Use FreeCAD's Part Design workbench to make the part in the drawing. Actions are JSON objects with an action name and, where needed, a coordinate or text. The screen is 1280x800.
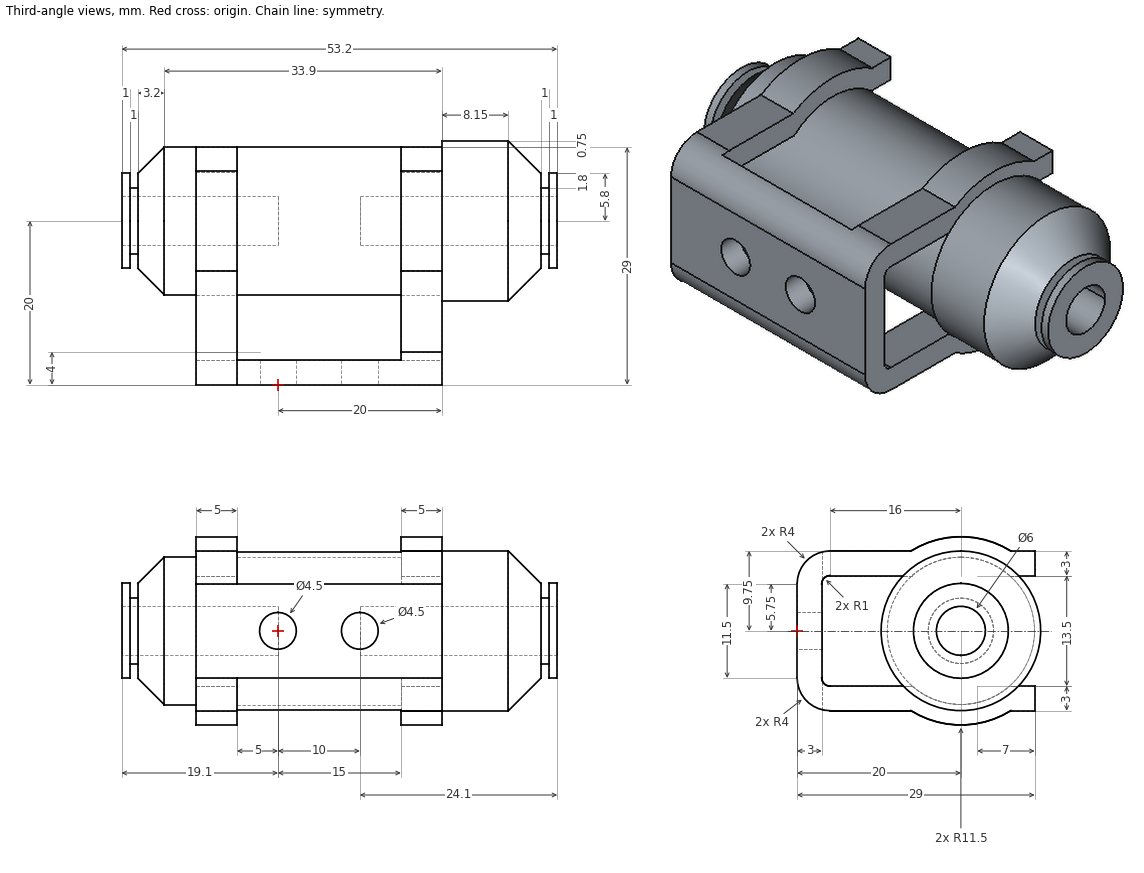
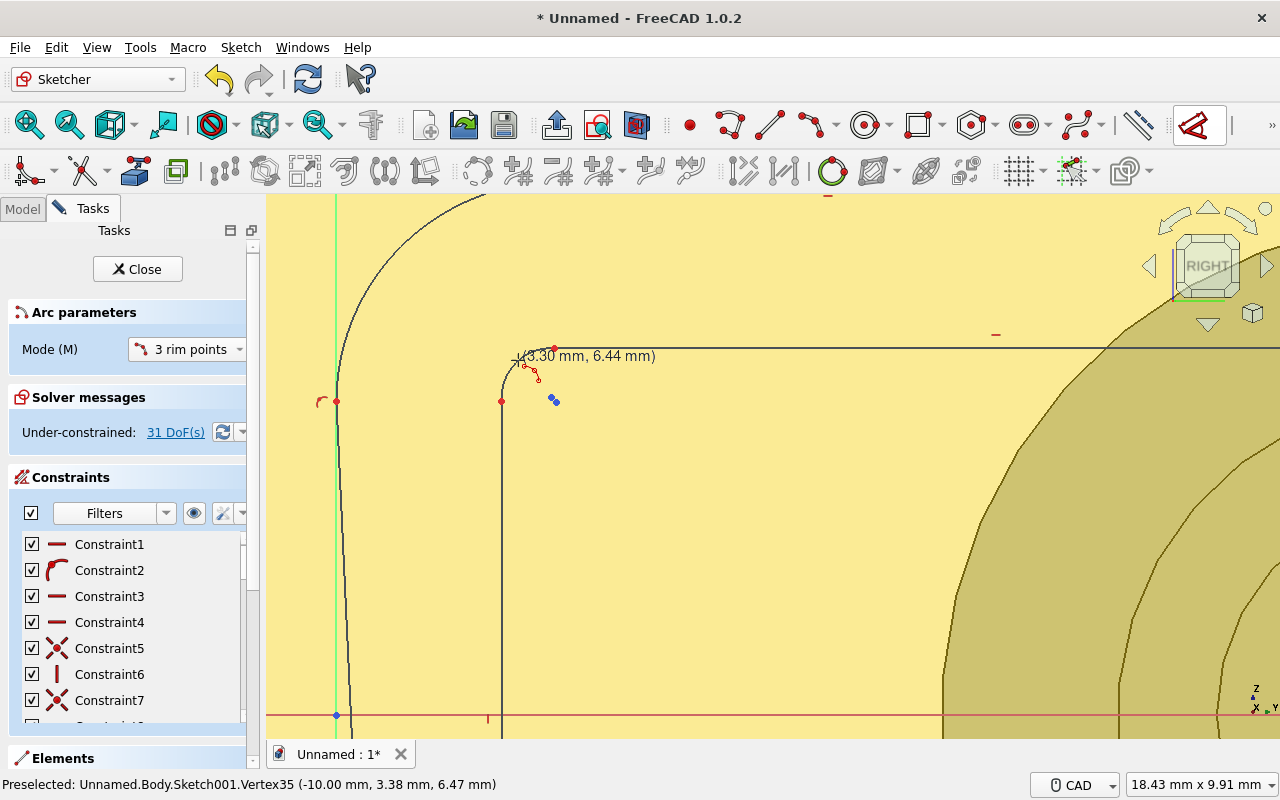
{"action": "scroll", "coordinate": [519, 359], "scroll_direction": "down", "scroll_amount": 6}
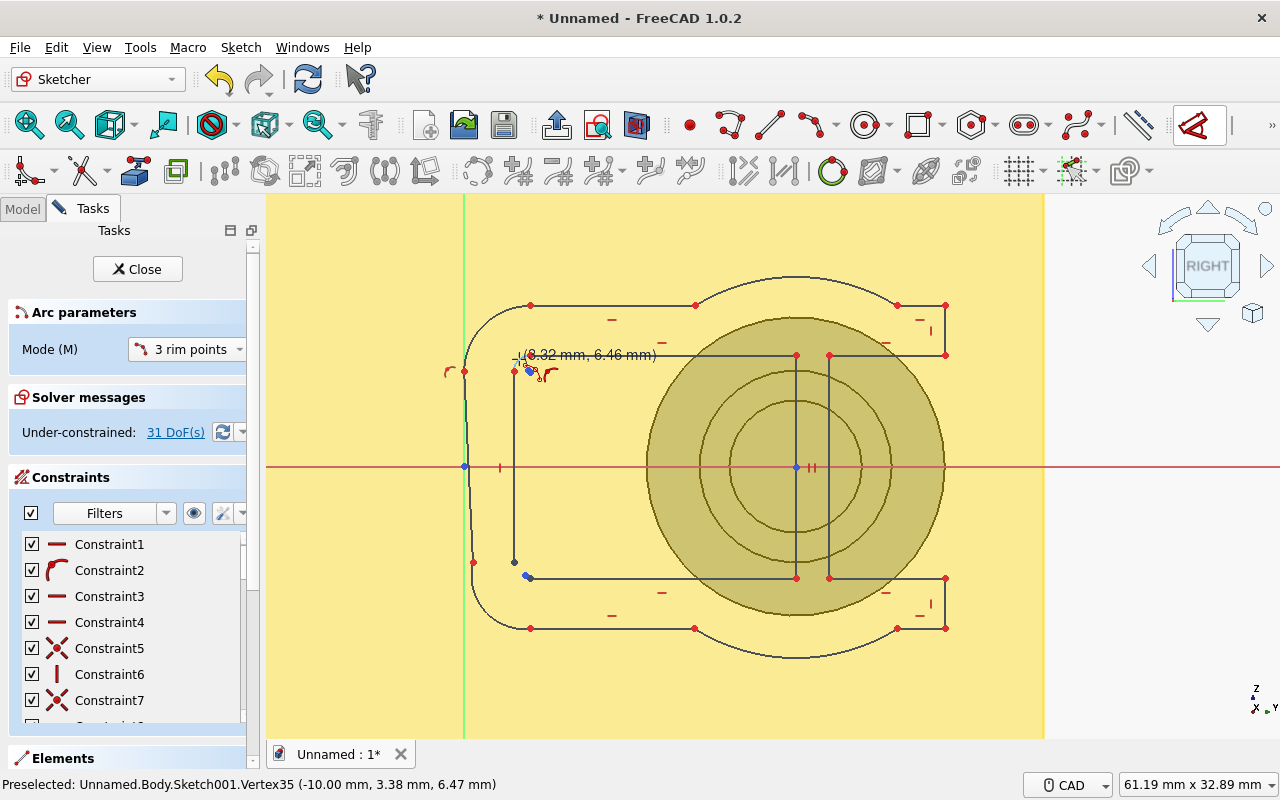
{"action": "left_click", "coordinate": [530, 579]}
{"action": "left_click", "coordinate": [514, 563]}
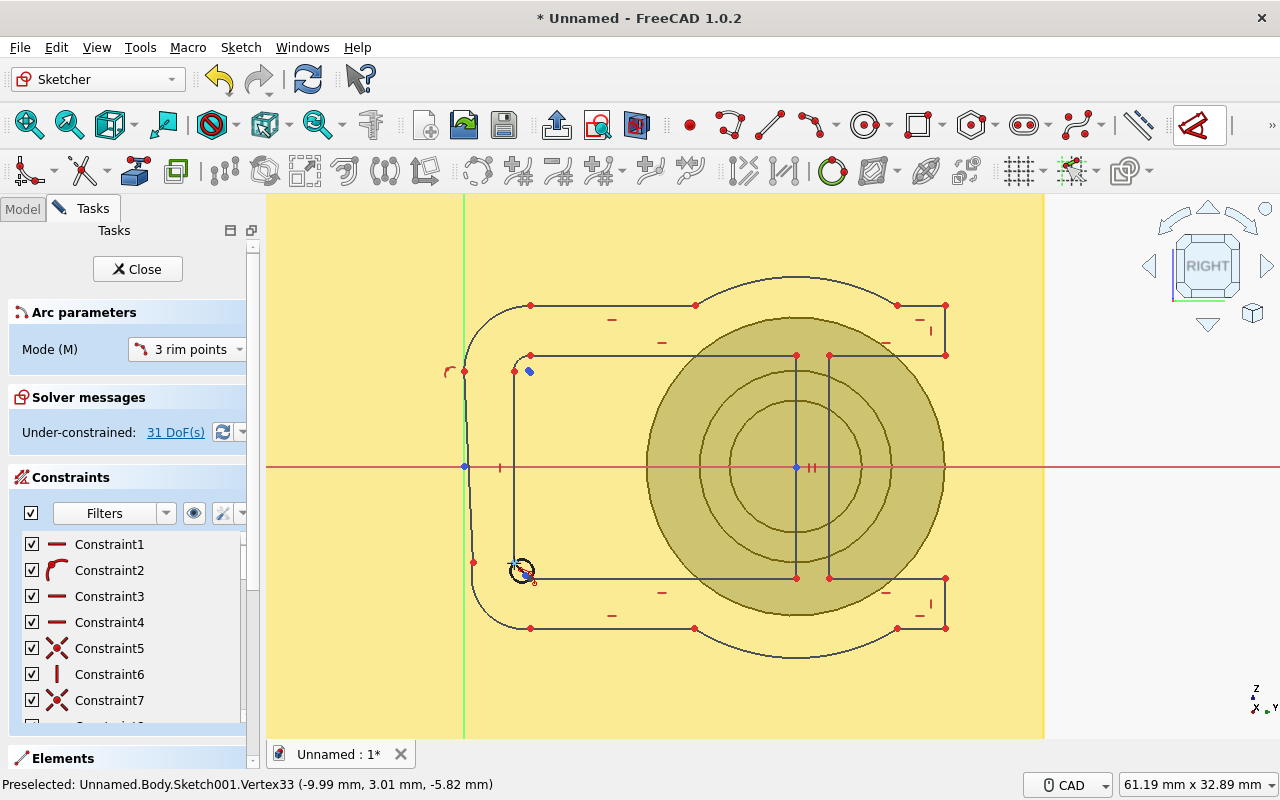
{"action": "scroll", "coordinate": [519, 574], "scroll_direction": "up", "scroll_amount": 6}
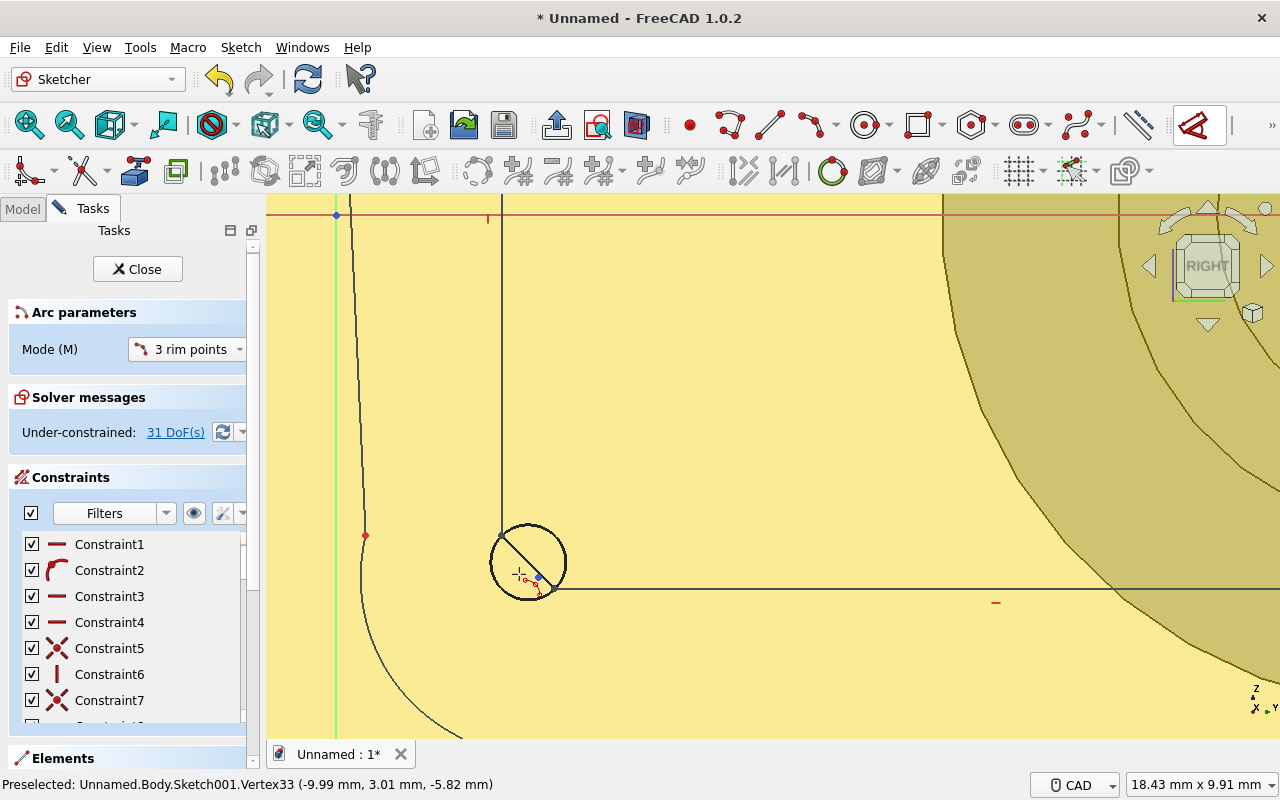
{"action": "left_click", "coordinate": [518, 571]}
{"action": "key", "text": "Escape"}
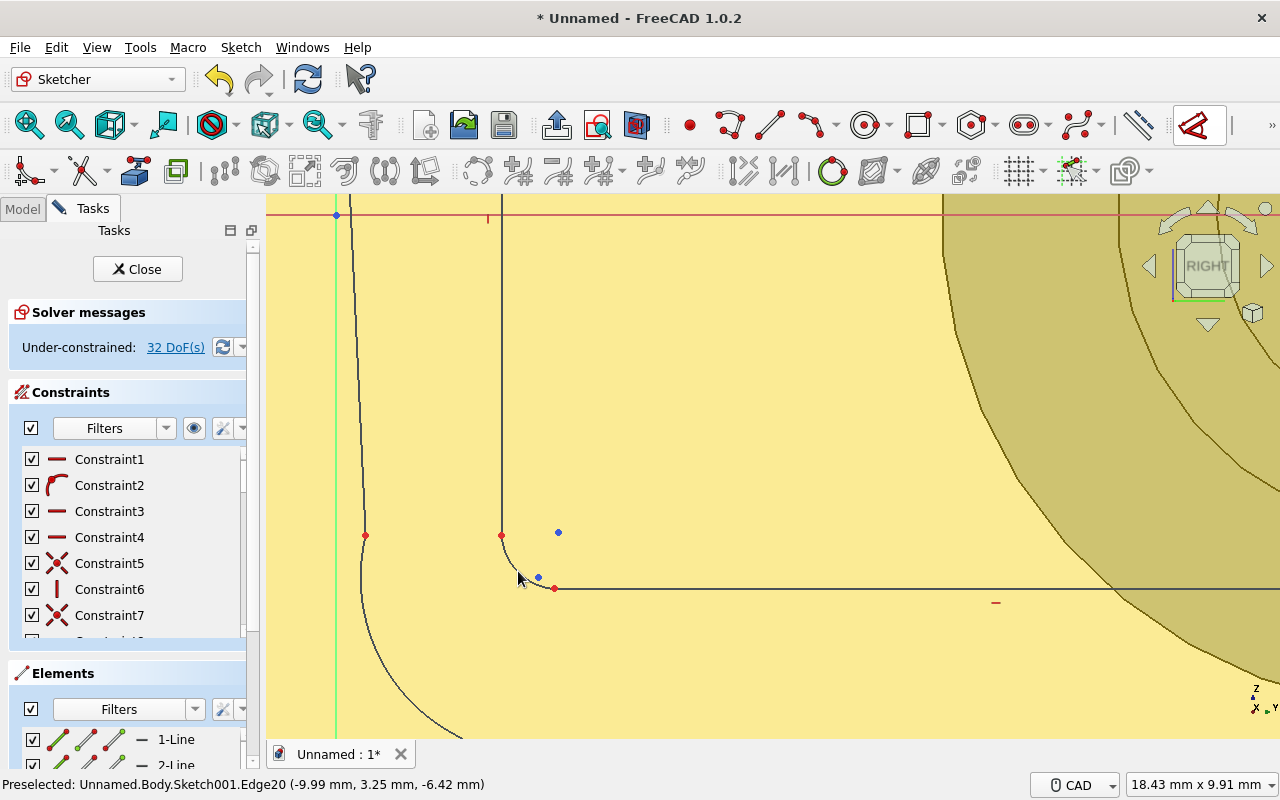
{"action": "scroll", "coordinate": [519, 575], "scroll_direction": "down", "scroll_amount": 6}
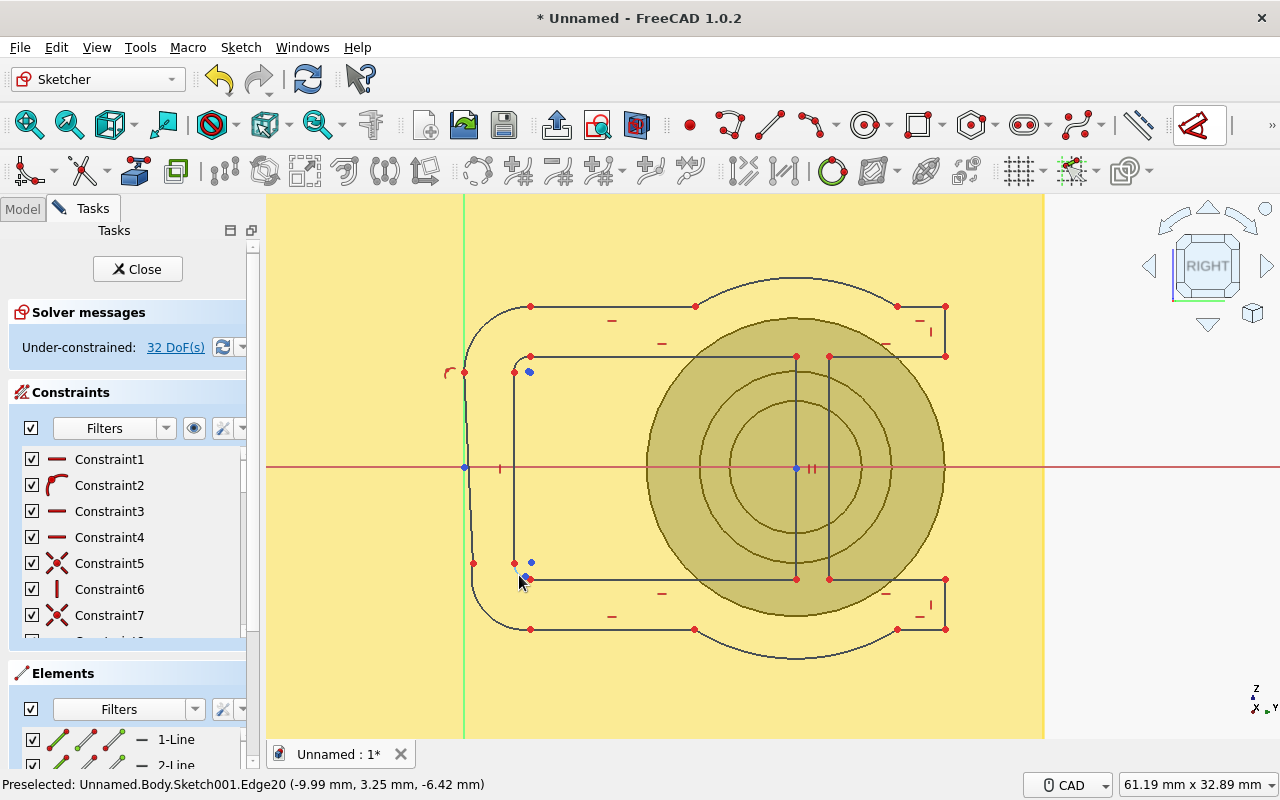
{"action": "left_click", "coordinate": [645, 307]}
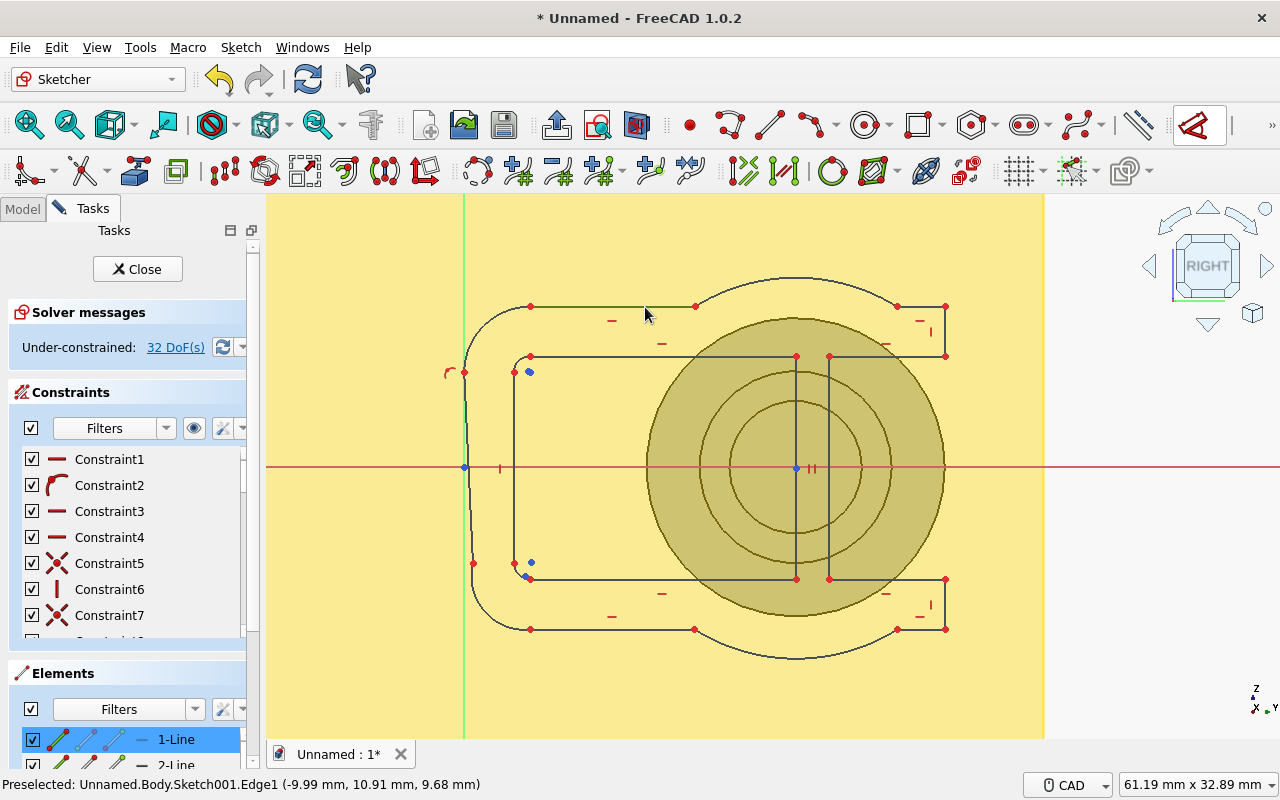
{"action": "left_click", "coordinate": [500, 314]}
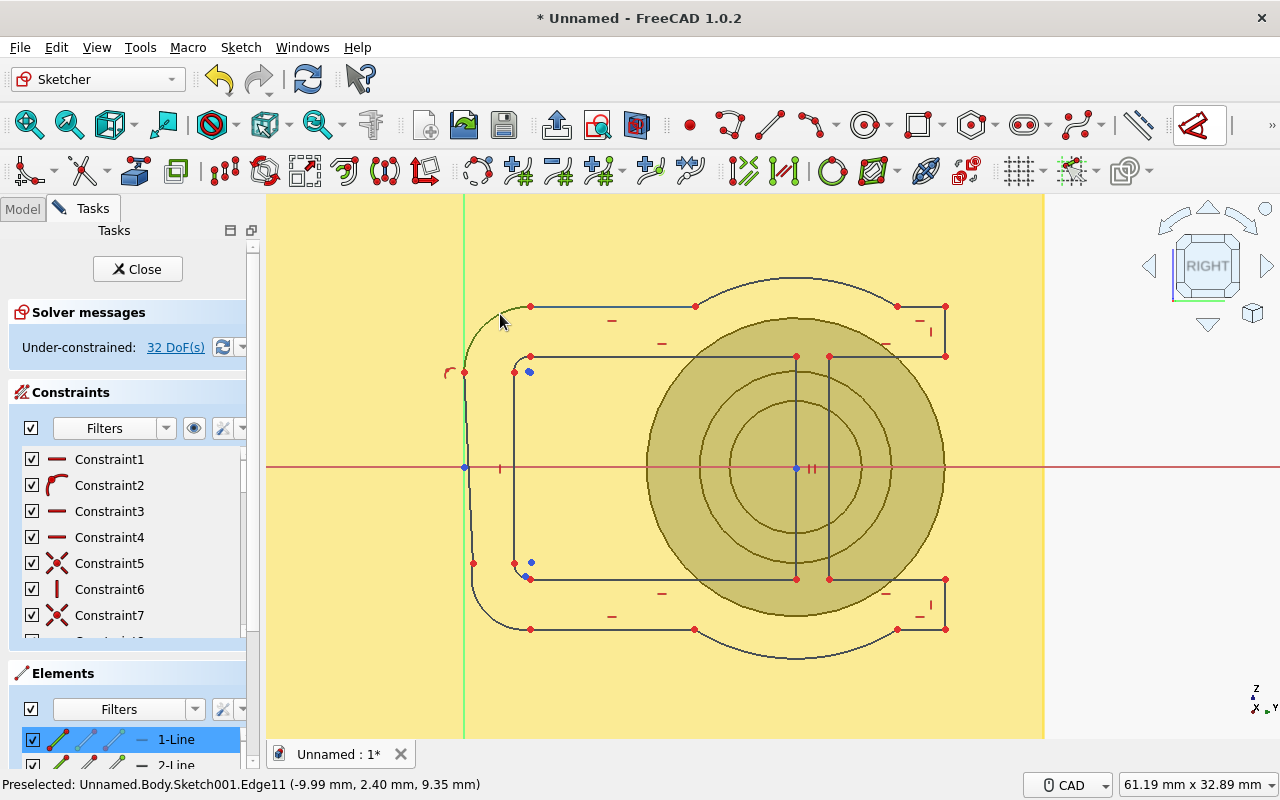
{"action": "key", "text": "t"}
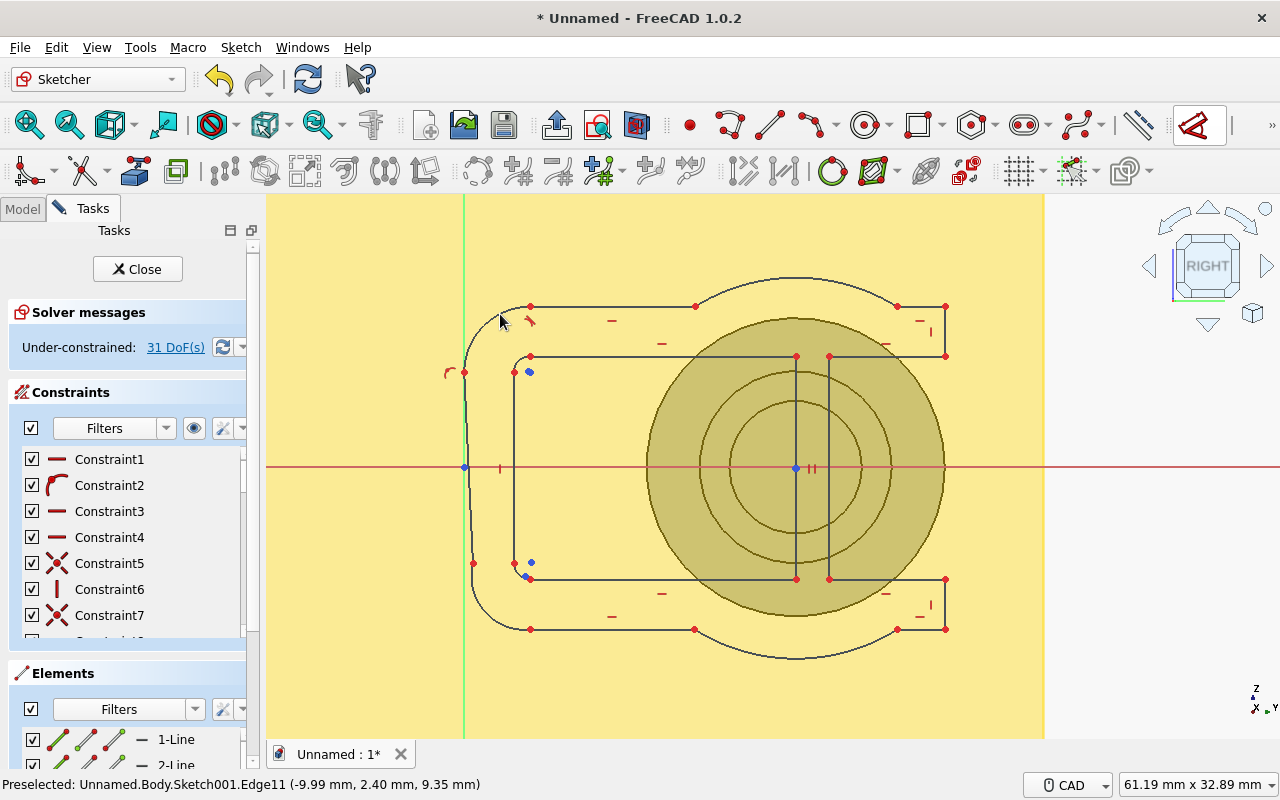
{"action": "left_click", "coordinate": [467, 430]}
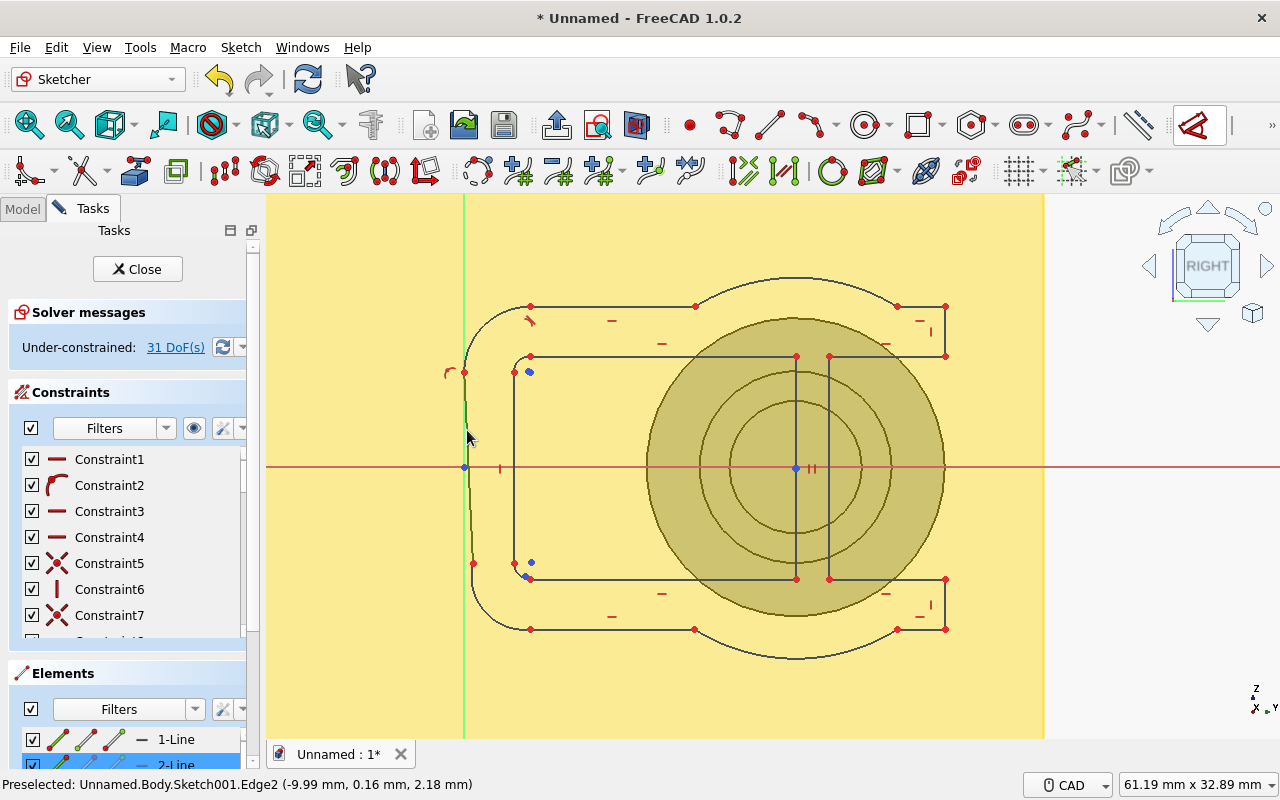
{"action": "left_click", "coordinate": [500, 314]}